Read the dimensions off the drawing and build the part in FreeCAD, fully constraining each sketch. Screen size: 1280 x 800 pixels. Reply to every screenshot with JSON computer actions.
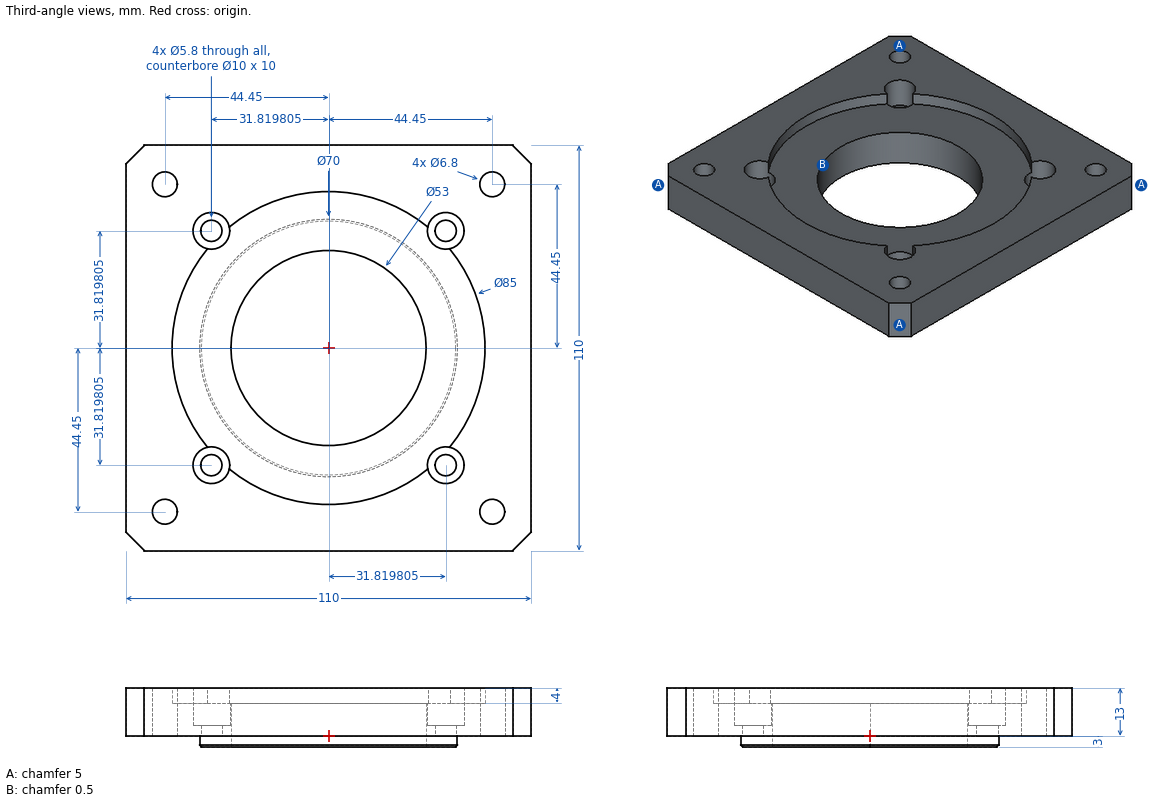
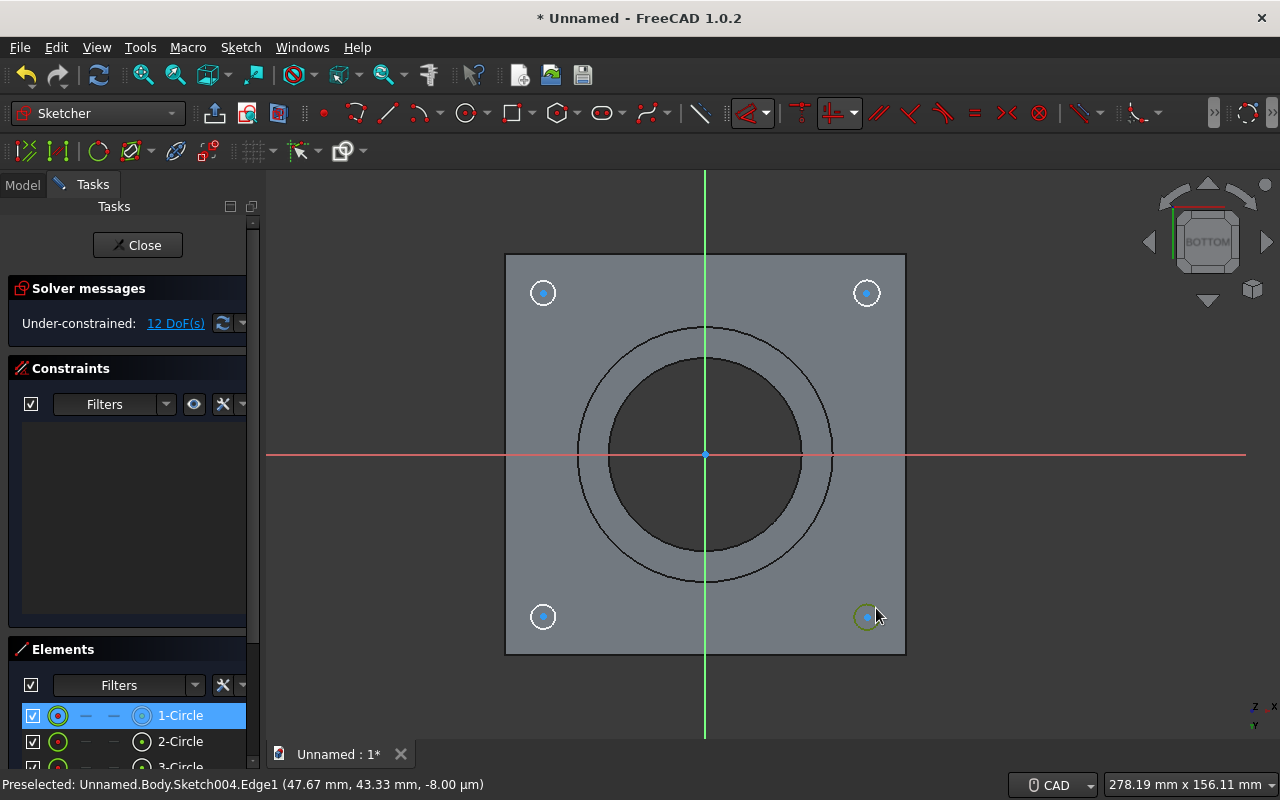
{"action": "left_click", "coordinate": [552, 608]}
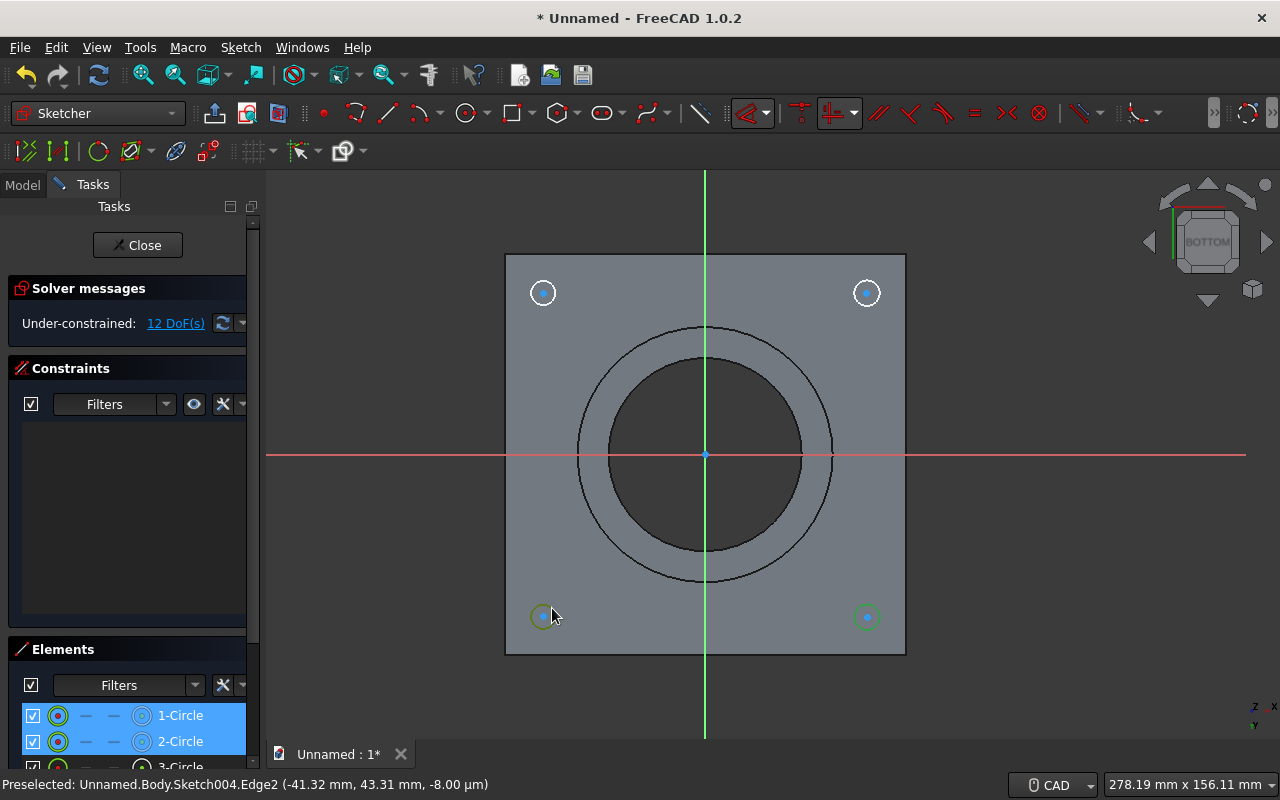
{"action": "left_click", "coordinate": [552, 284]}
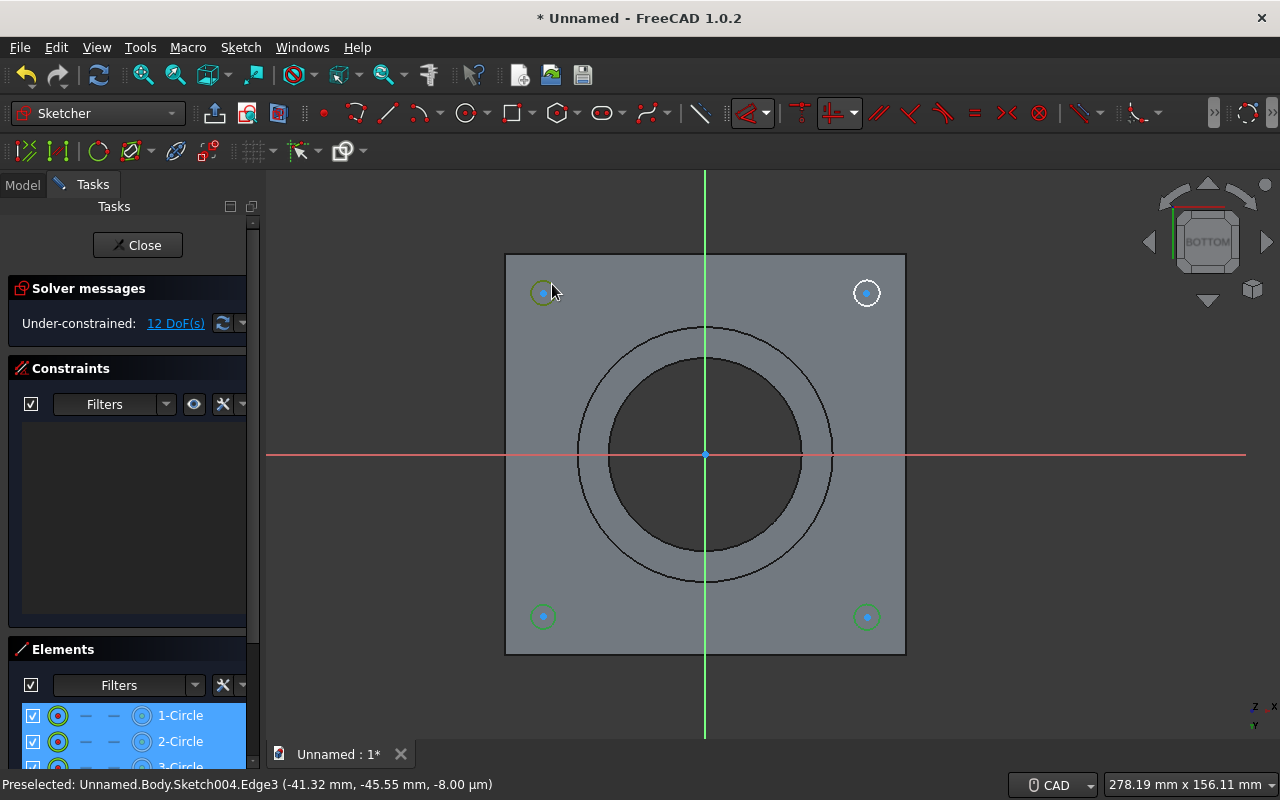
{"action": "left_click", "coordinate": [876, 284]}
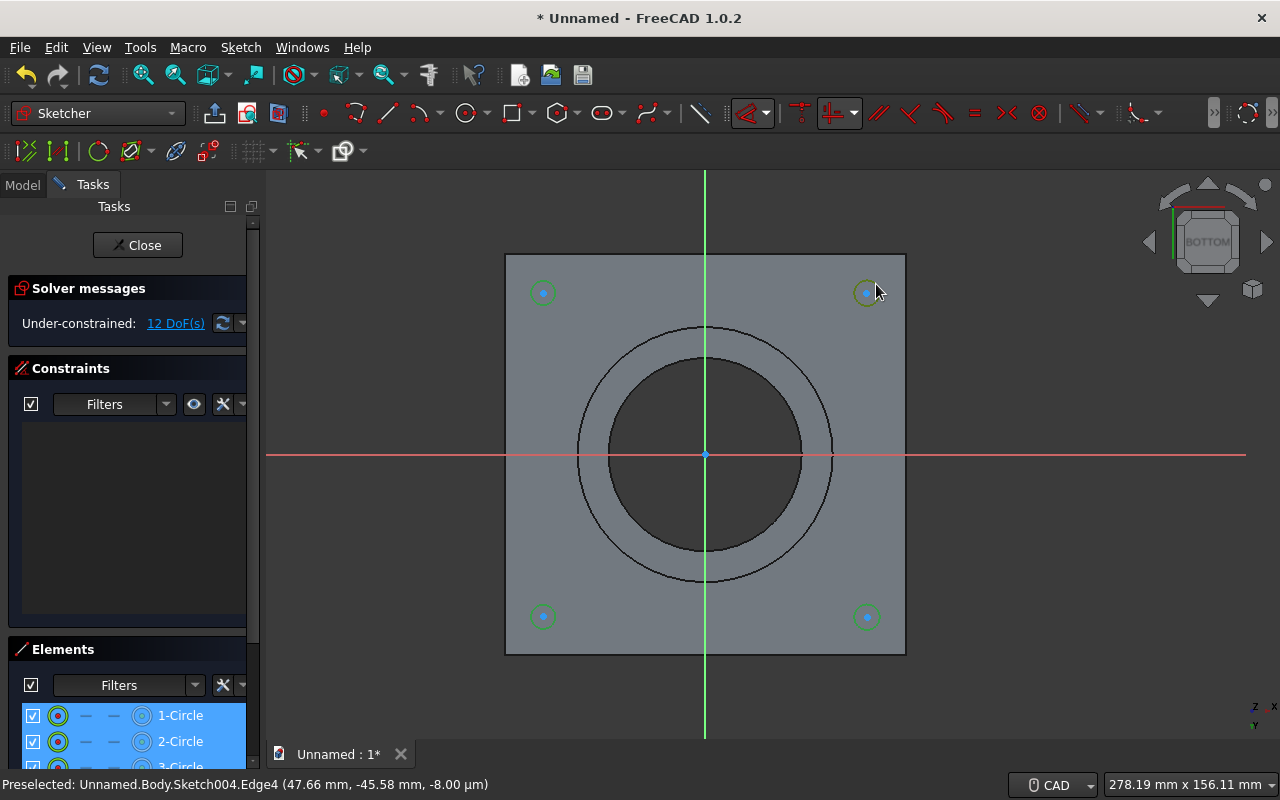
{"action": "key", "text": "e"}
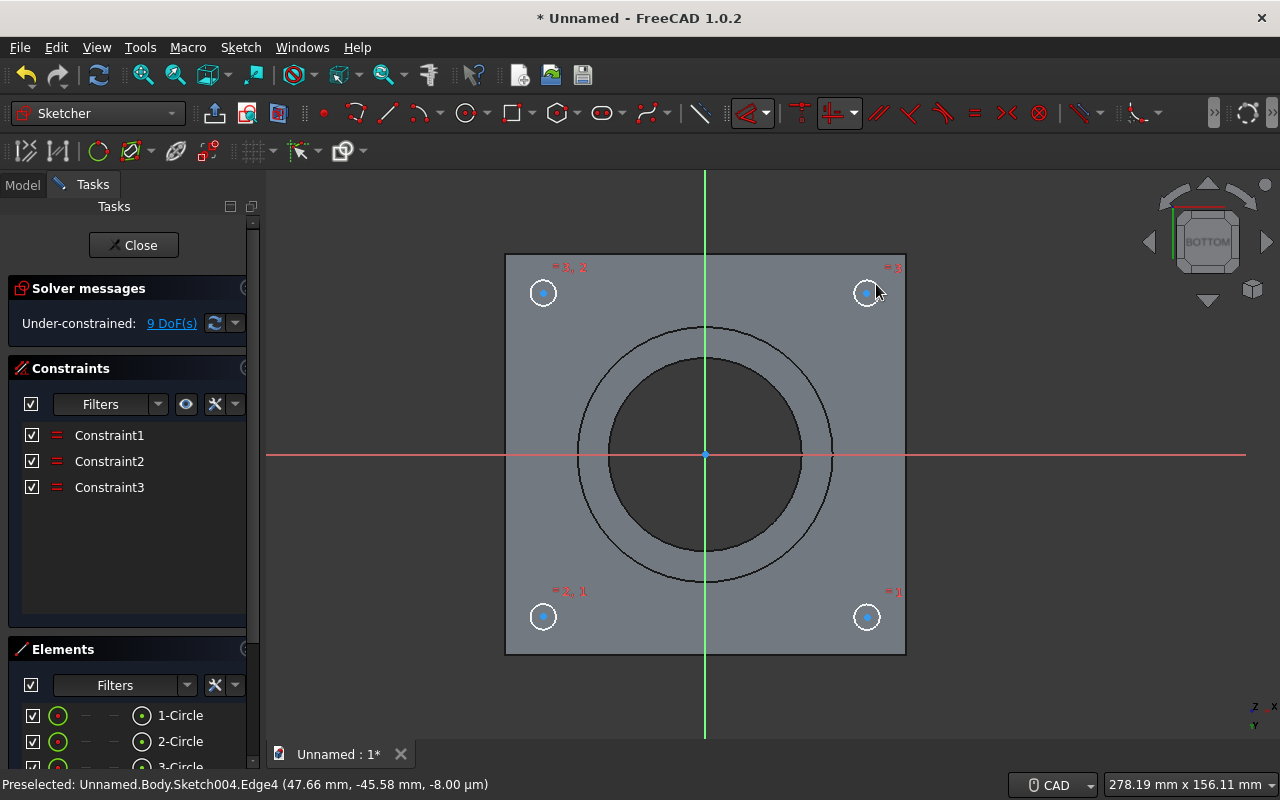
{"action": "left_click", "coordinate": [867, 617]}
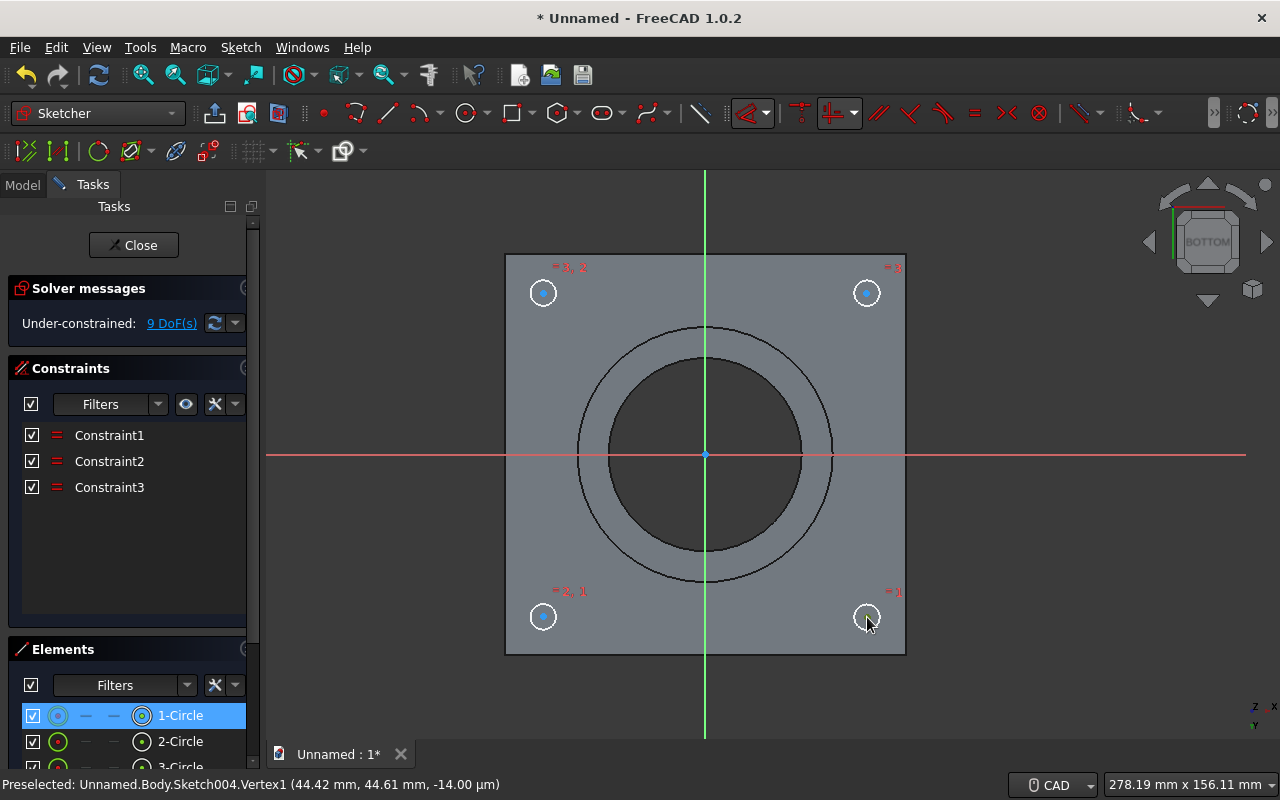
{"action": "left_click", "coordinate": [543, 617]}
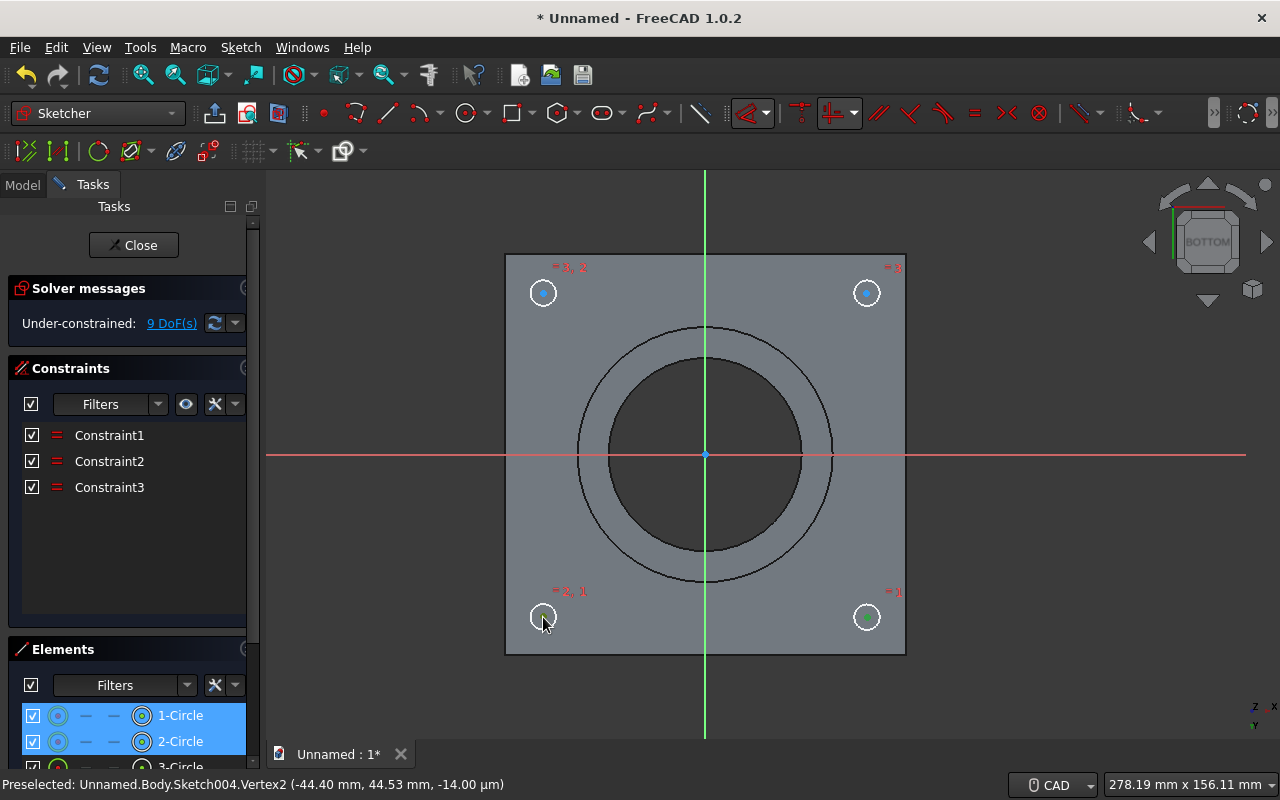
{"action": "key", "text": "h"}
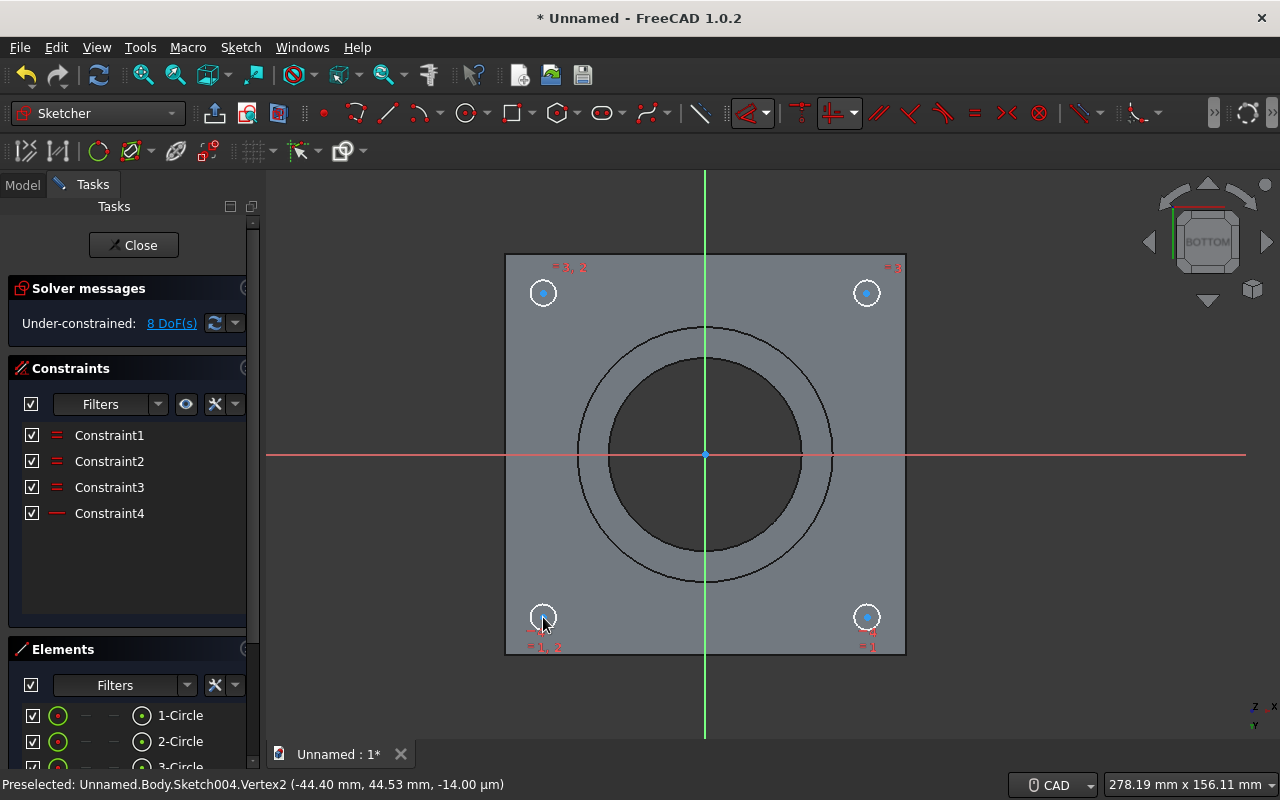
{"action": "left_click", "coordinate": [543, 617]}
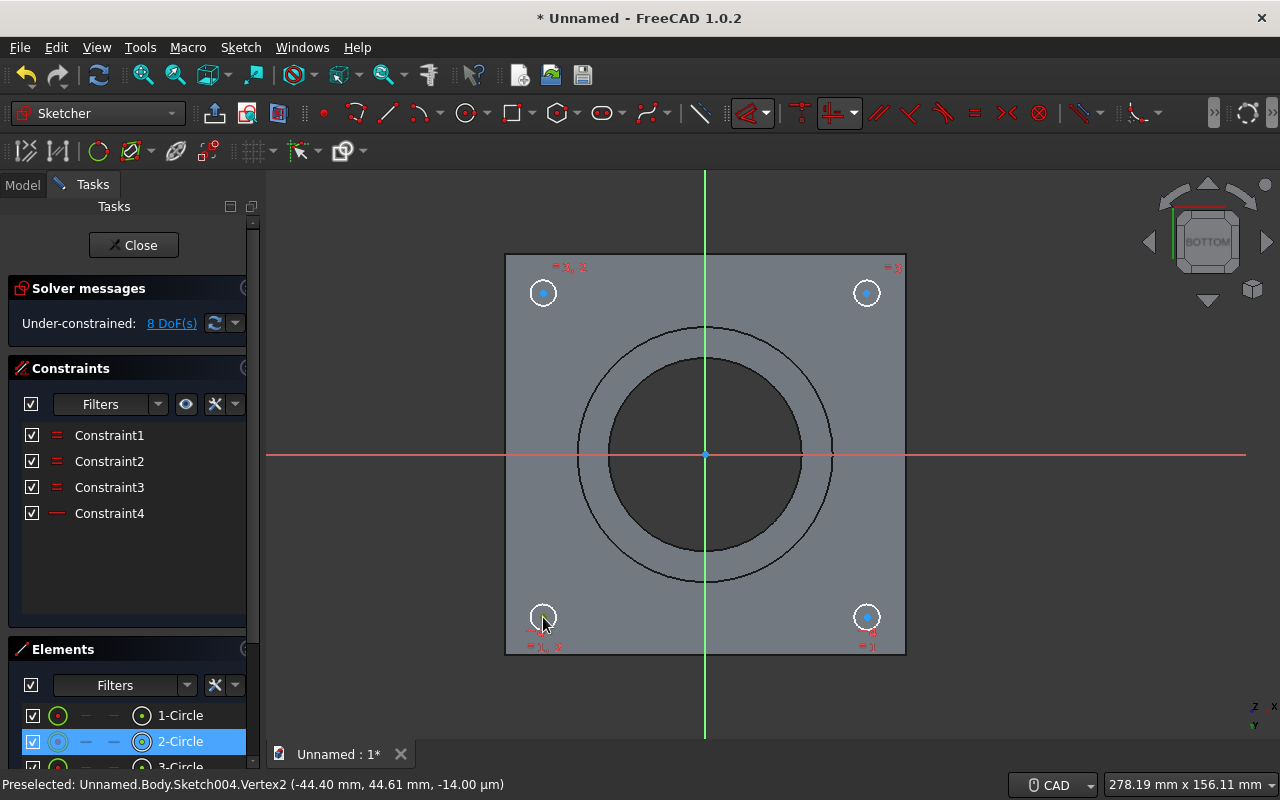
{"action": "left_click", "coordinate": [543, 293]}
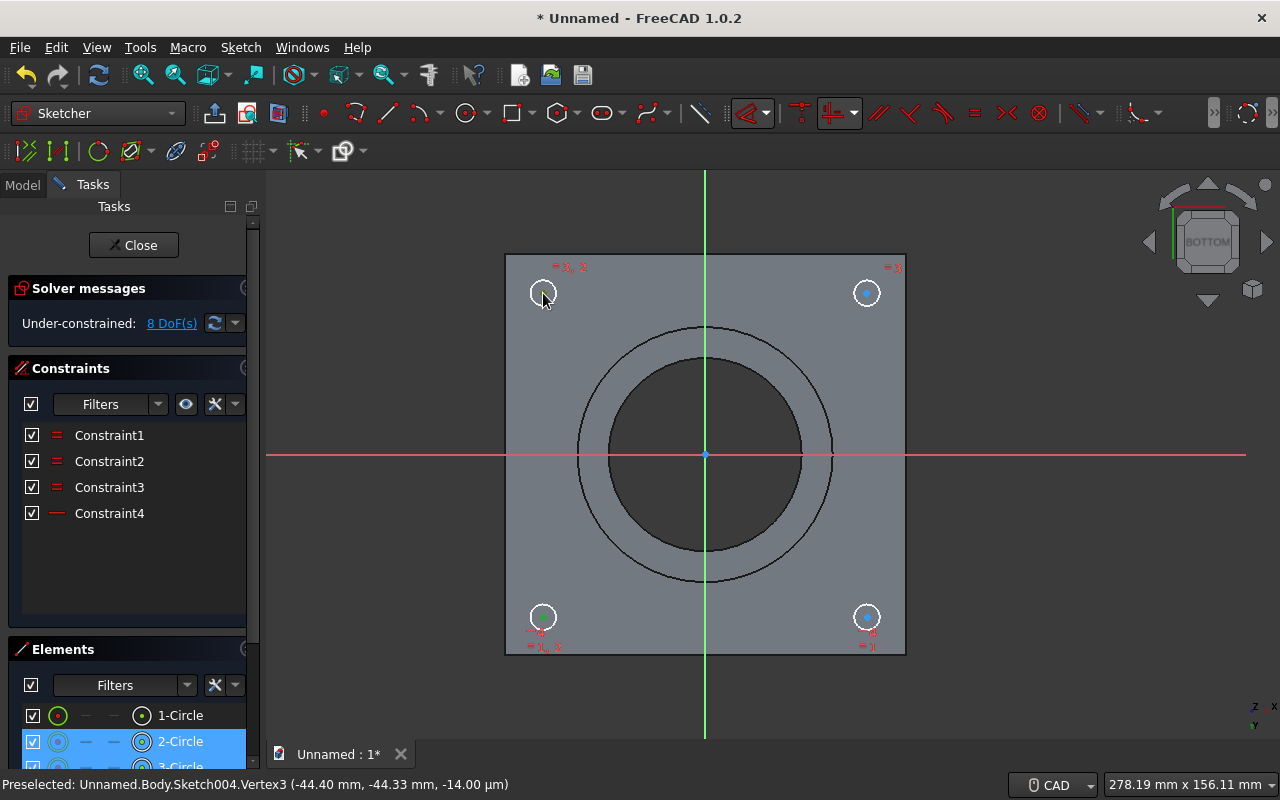
{"action": "key", "text": "v"}